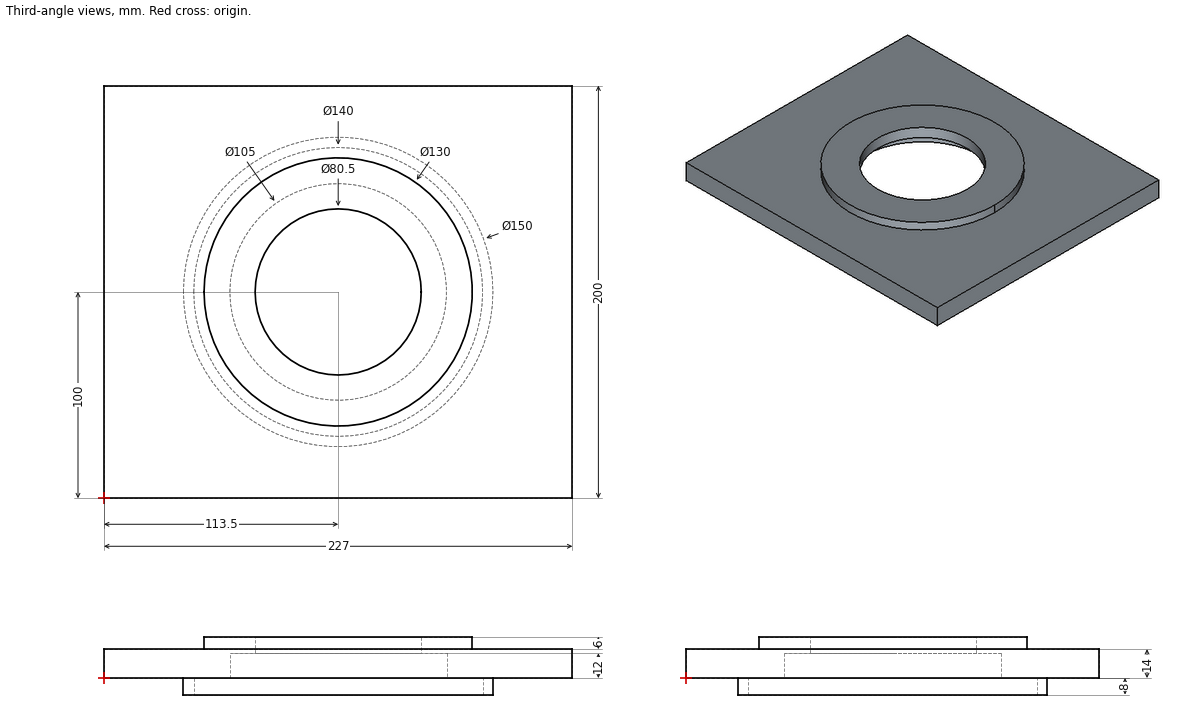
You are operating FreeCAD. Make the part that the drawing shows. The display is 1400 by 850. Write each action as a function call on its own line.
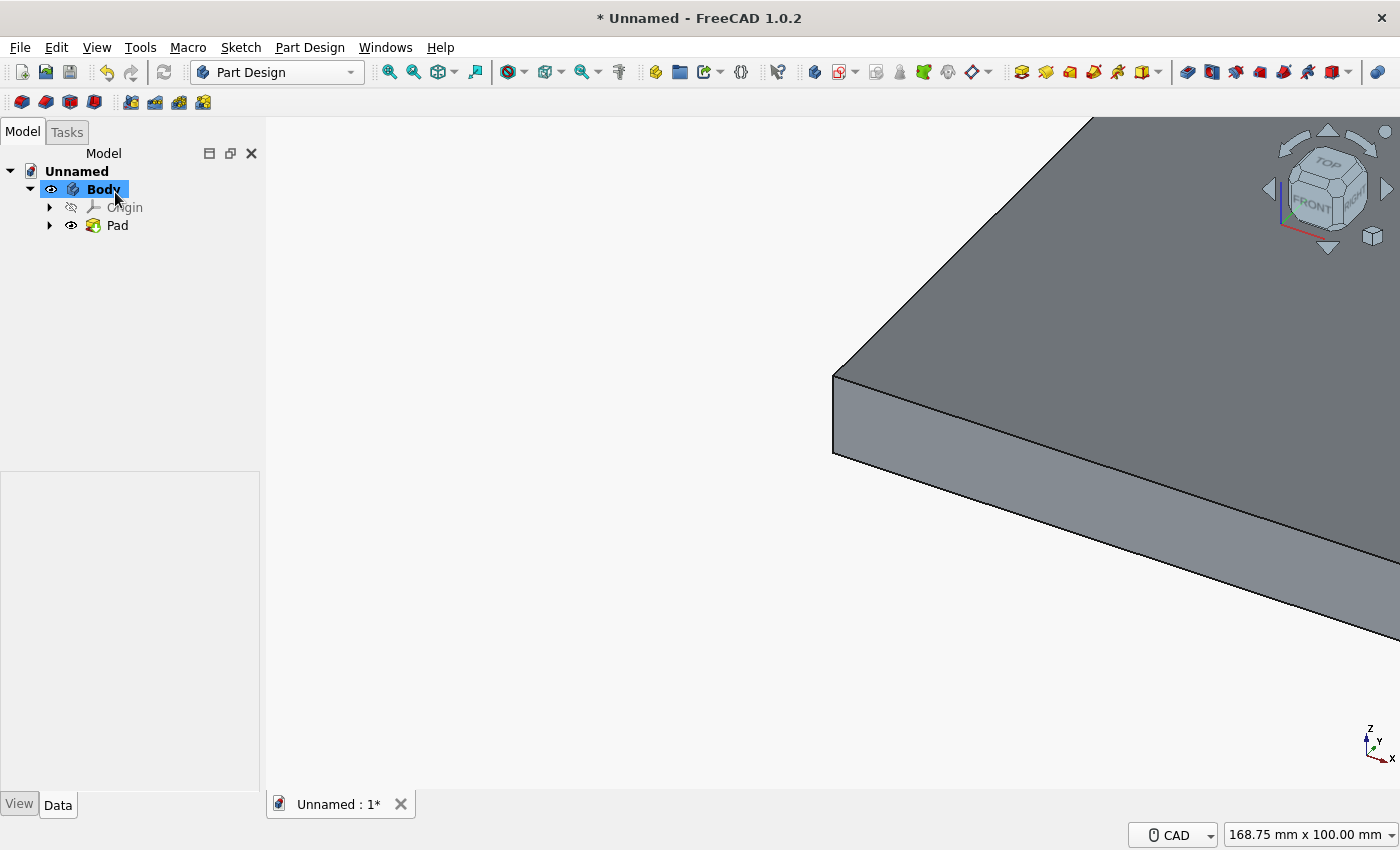
click(390, 72)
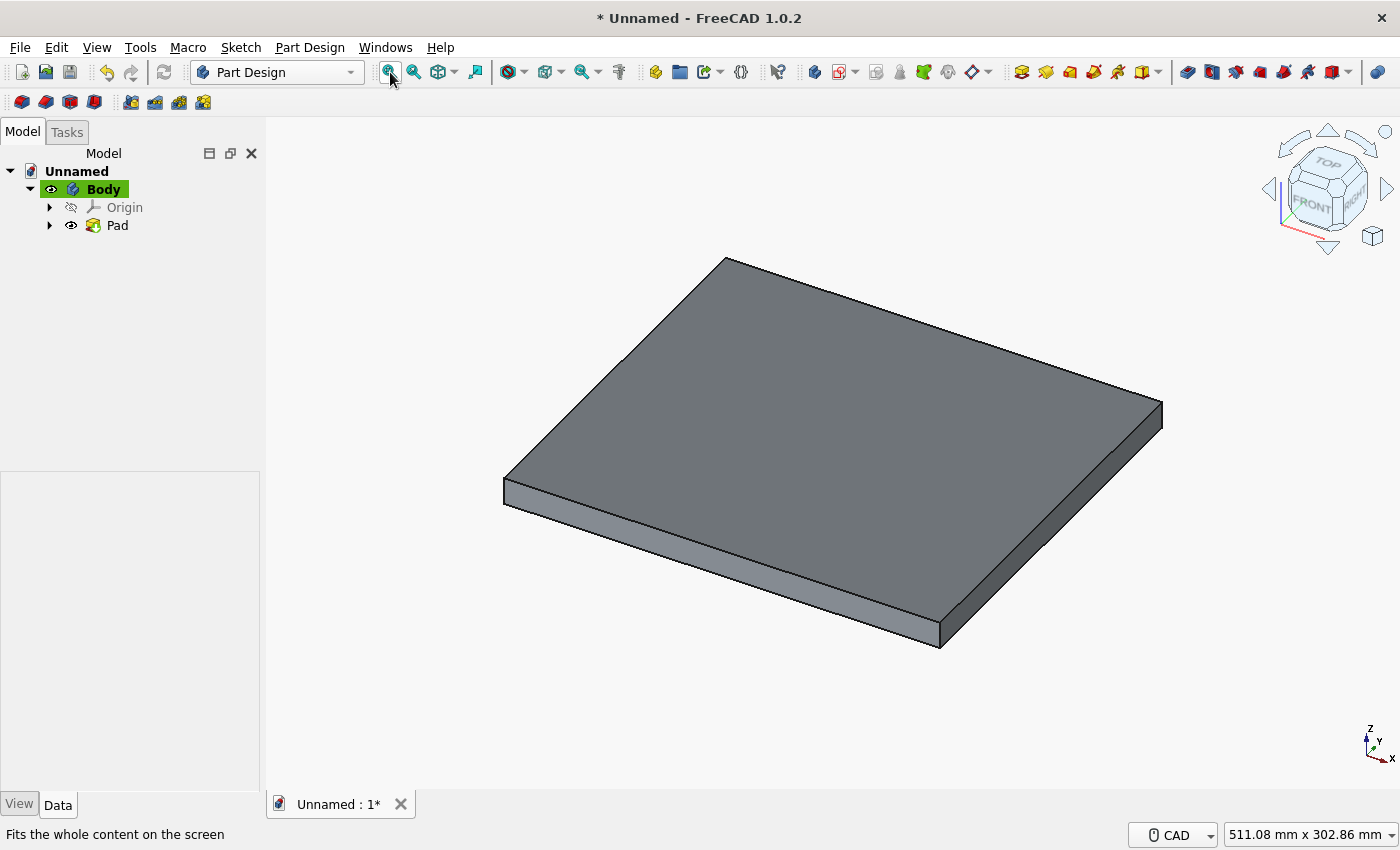
click(833, 439)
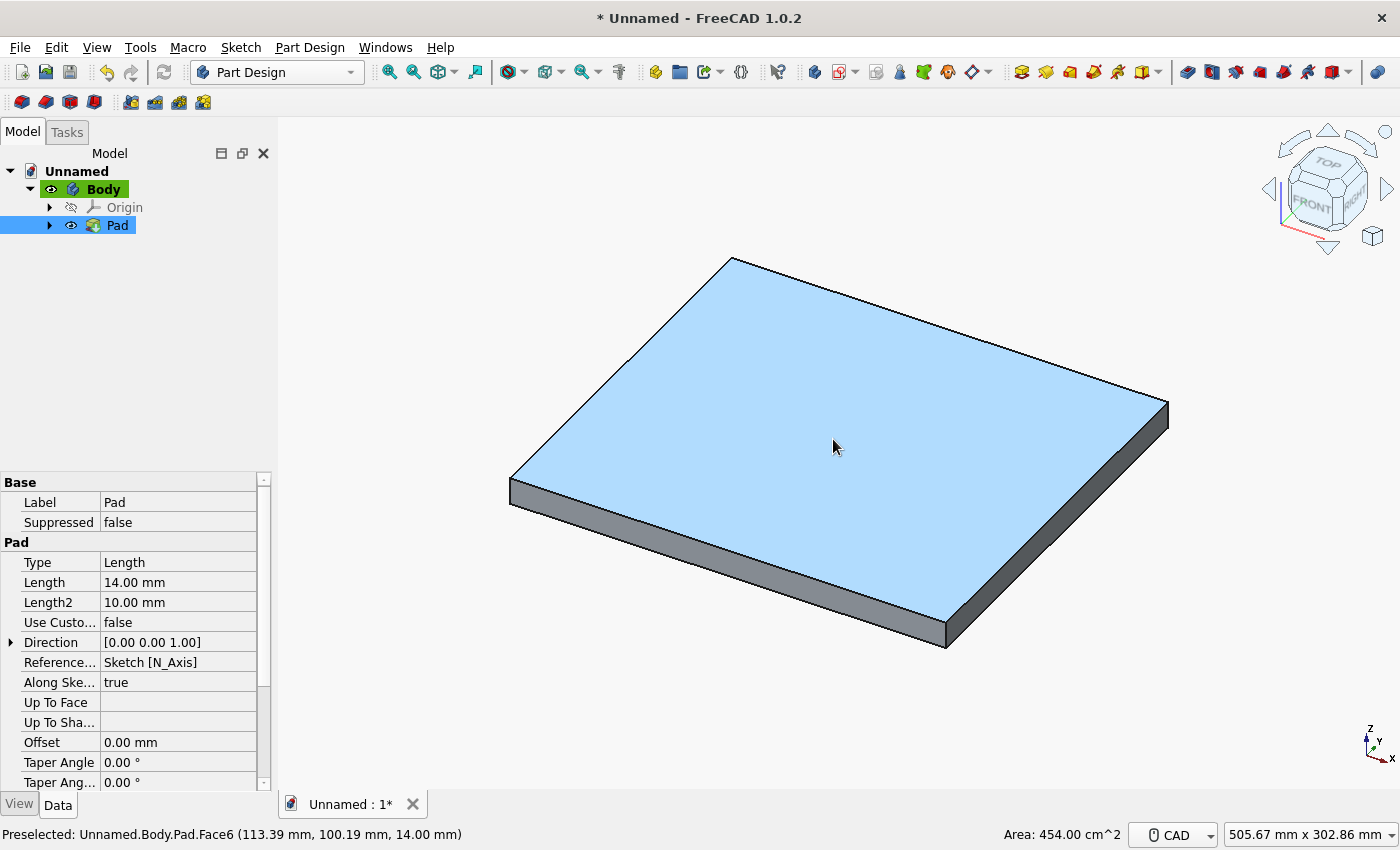
click(840, 72)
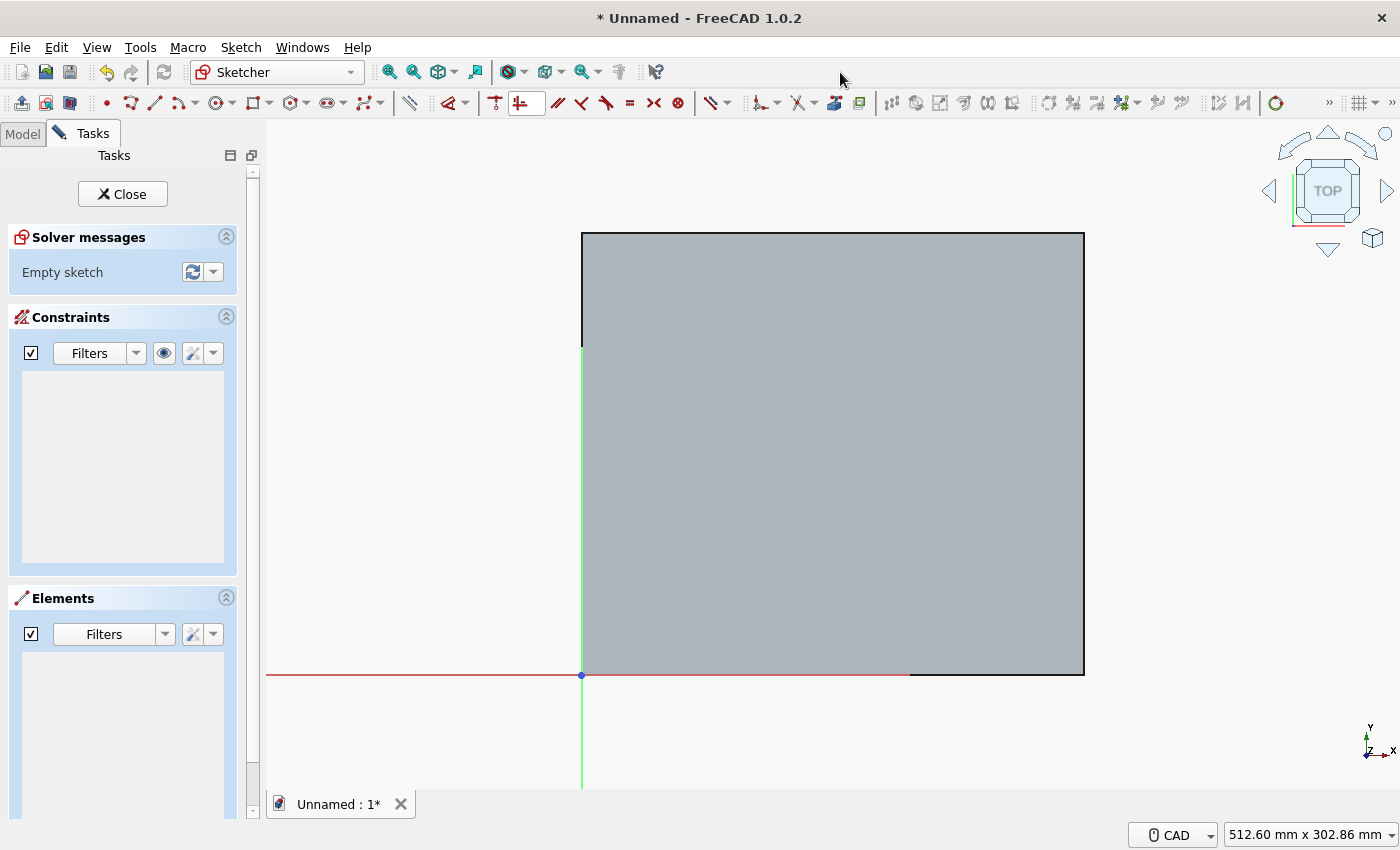
key(g)
key(c)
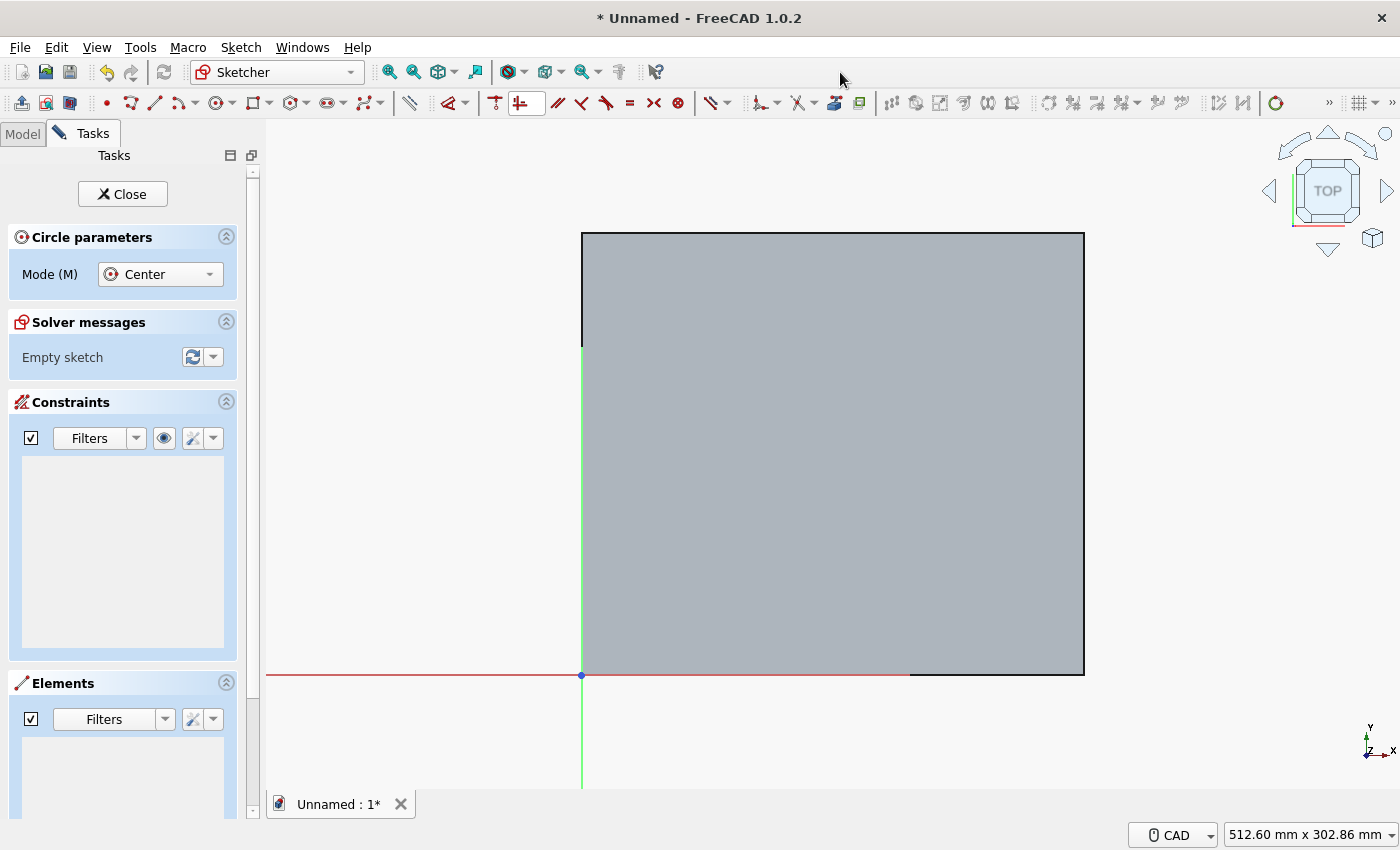
click(833, 454)
click(935, 352)
key(Escape)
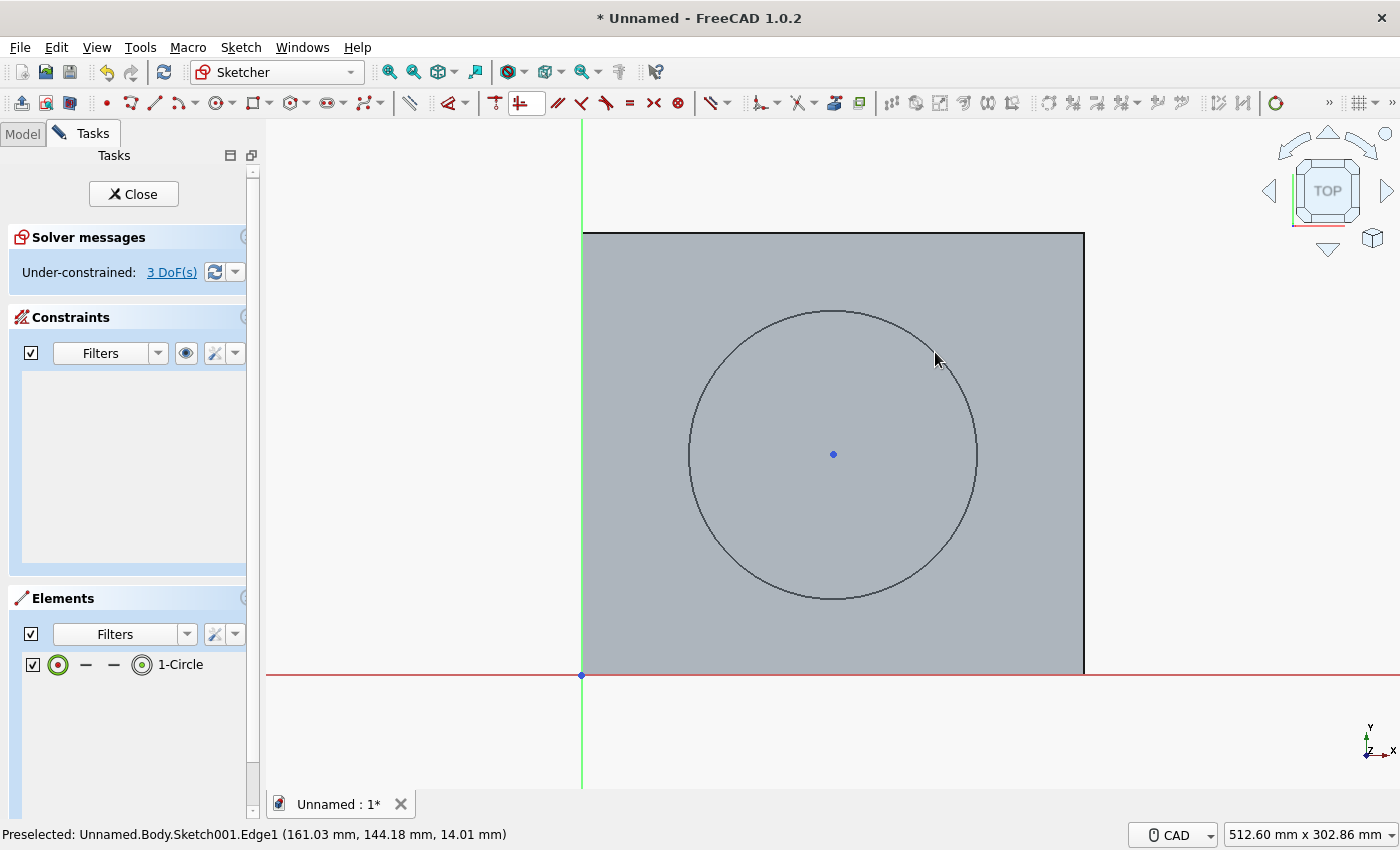
click(448, 104)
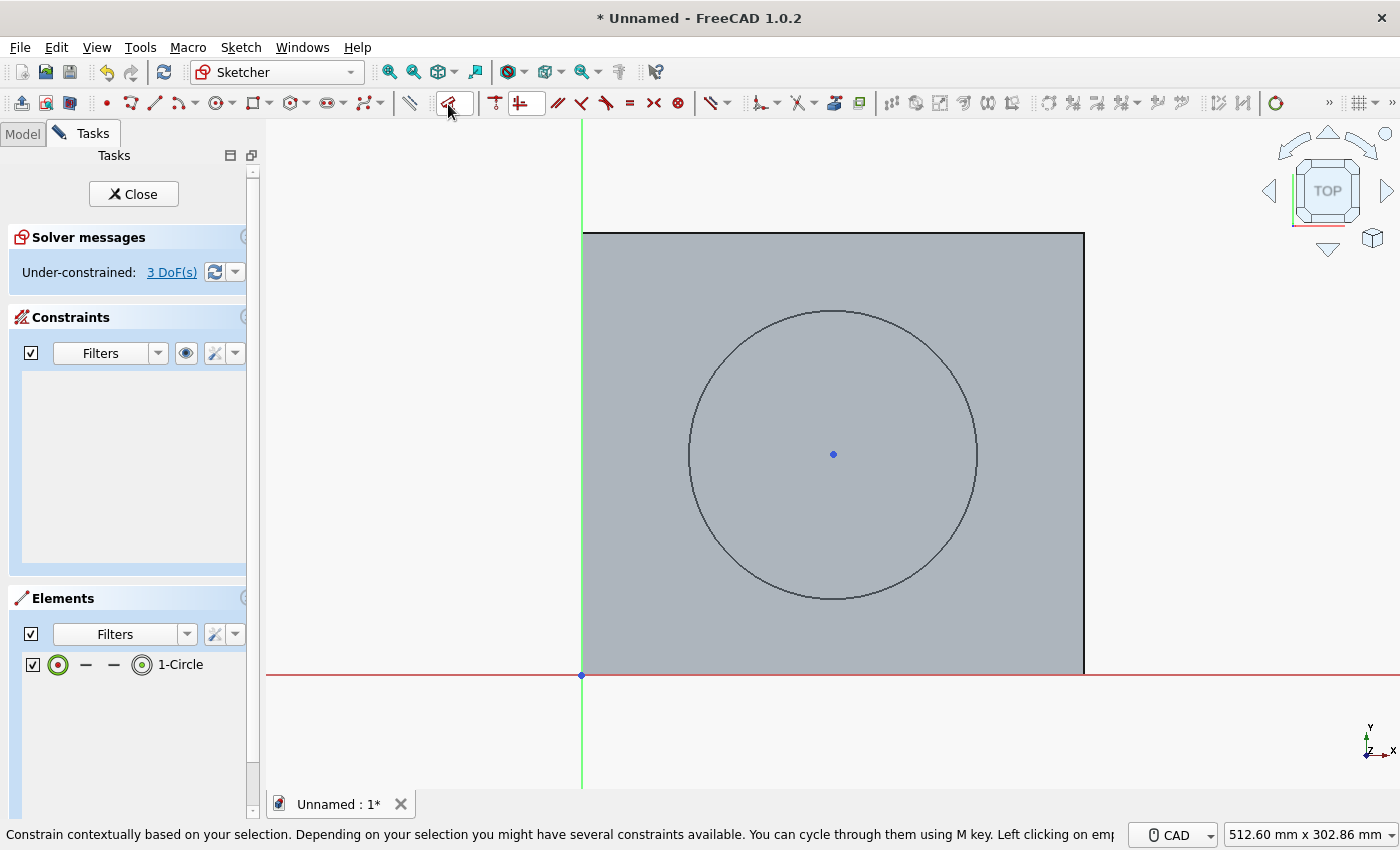
click(935, 353)
click(958, 330)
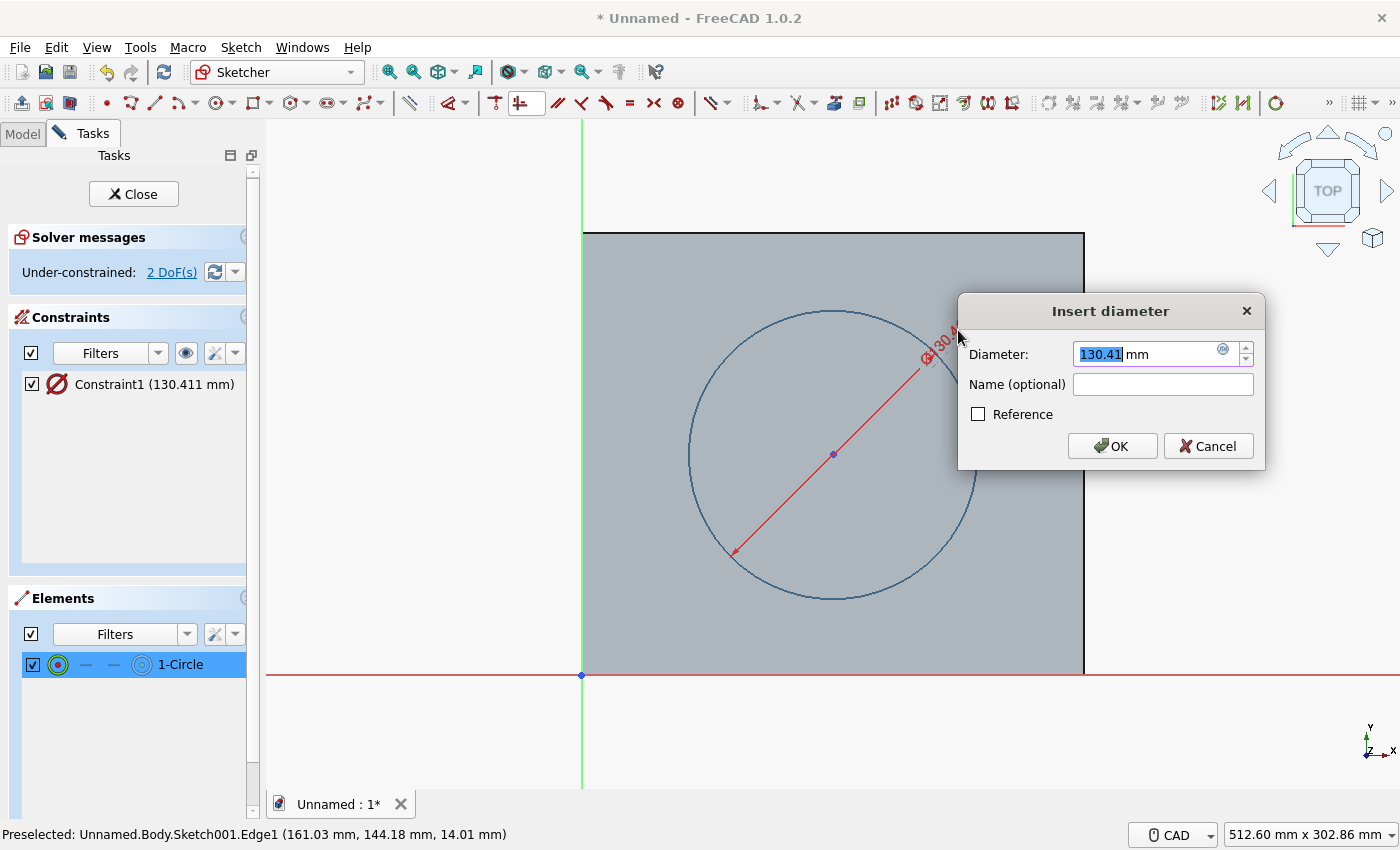
text(130)
key(Return)